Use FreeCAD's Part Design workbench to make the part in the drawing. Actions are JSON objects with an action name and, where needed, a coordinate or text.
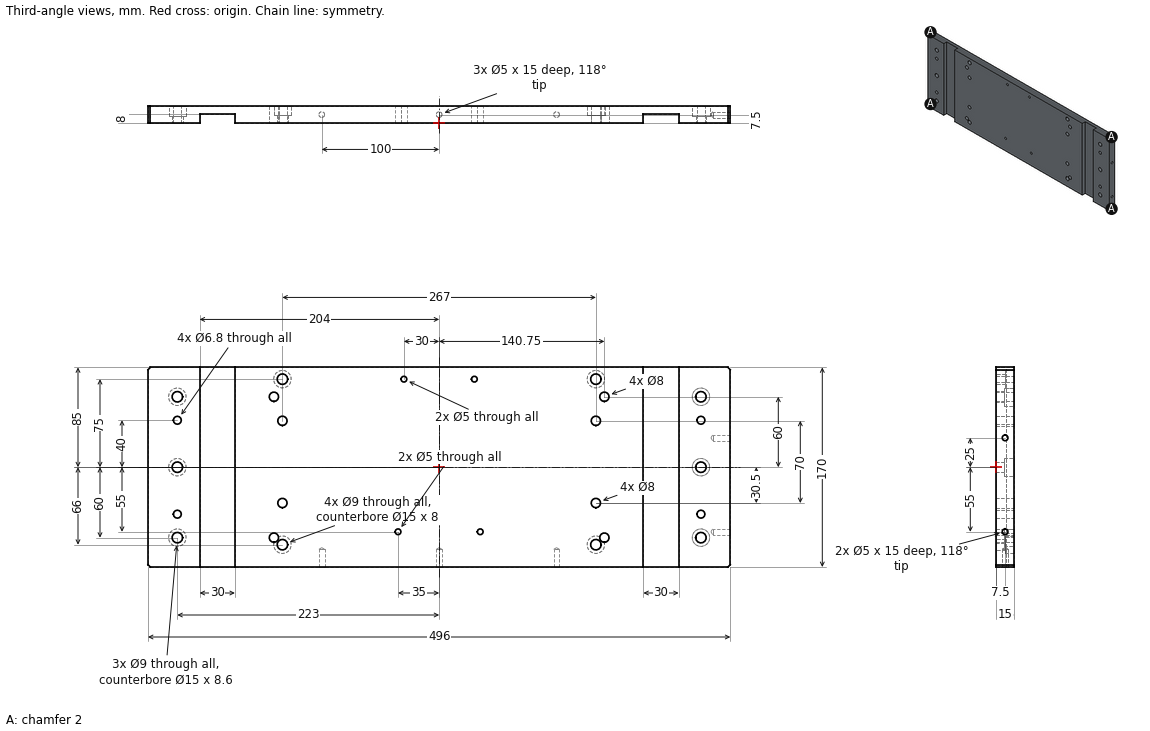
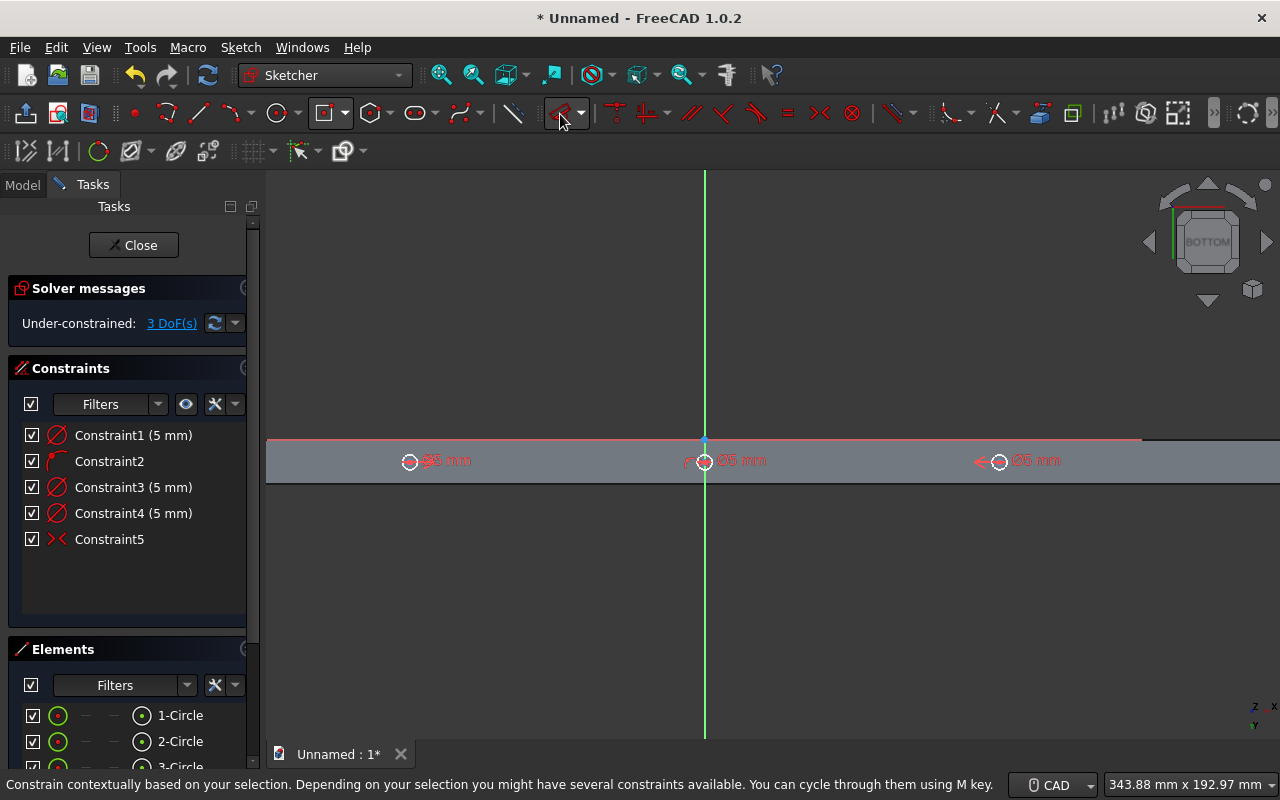
{"action": "scroll", "coordinate": [705, 462], "scroll_direction": "up", "scroll_amount": 3}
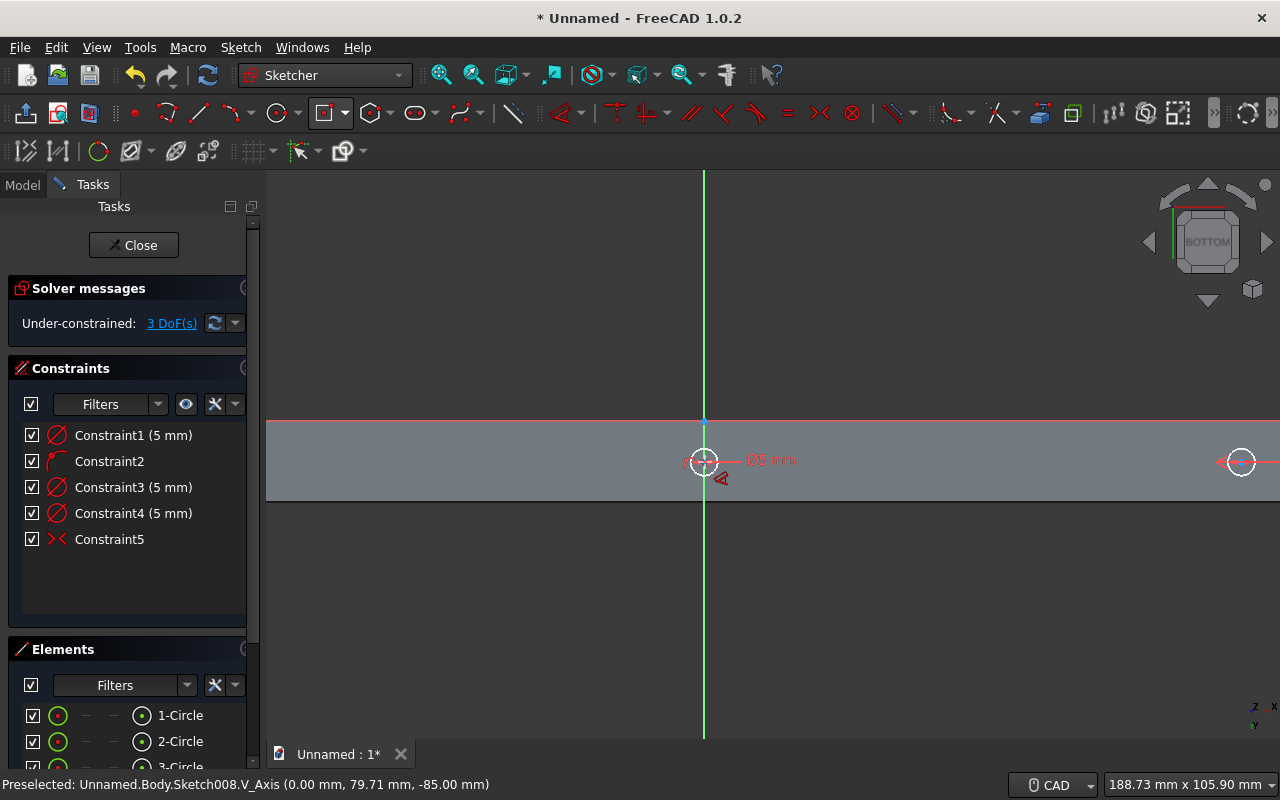
{"action": "left_click", "coordinate": [704, 462]}
{"action": "left_click", "coordinate": [738, 442]}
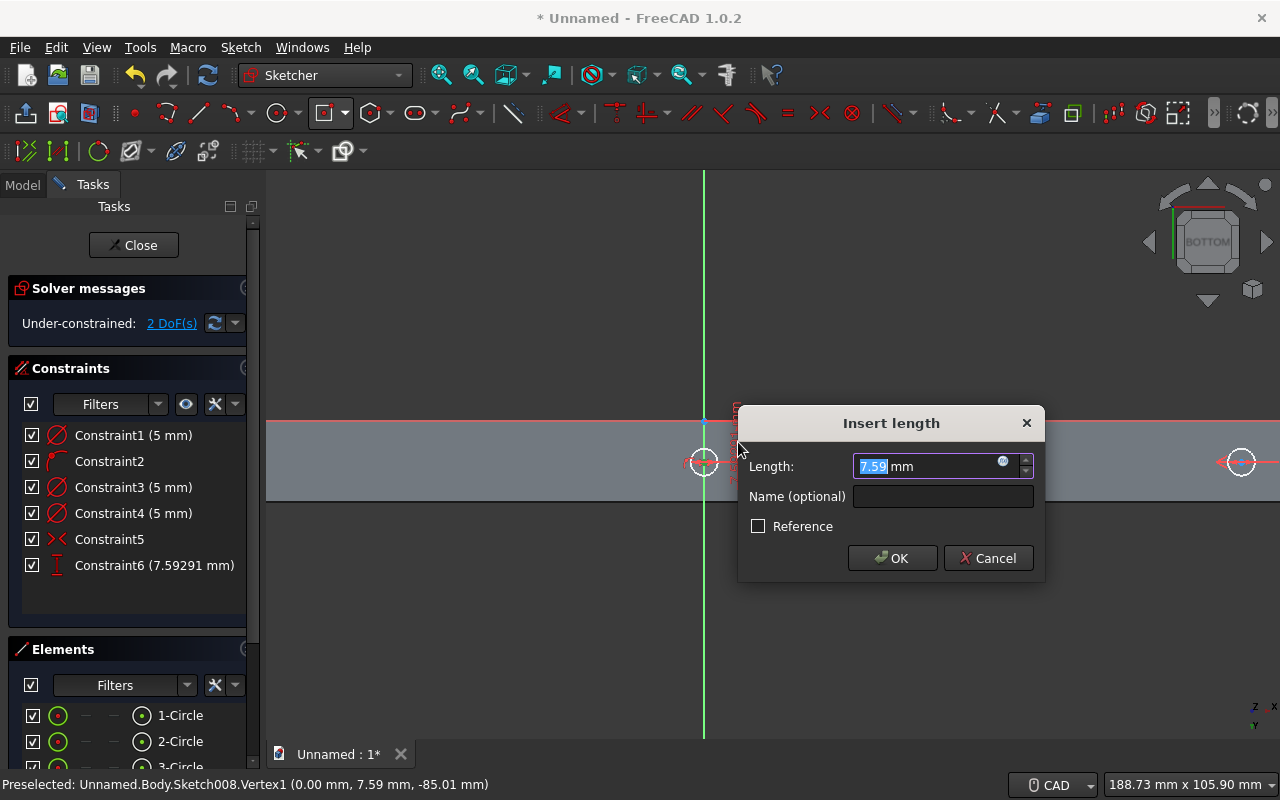
{"action": "type", "text": "7.5"}
{"action": "key", "text": "Return"}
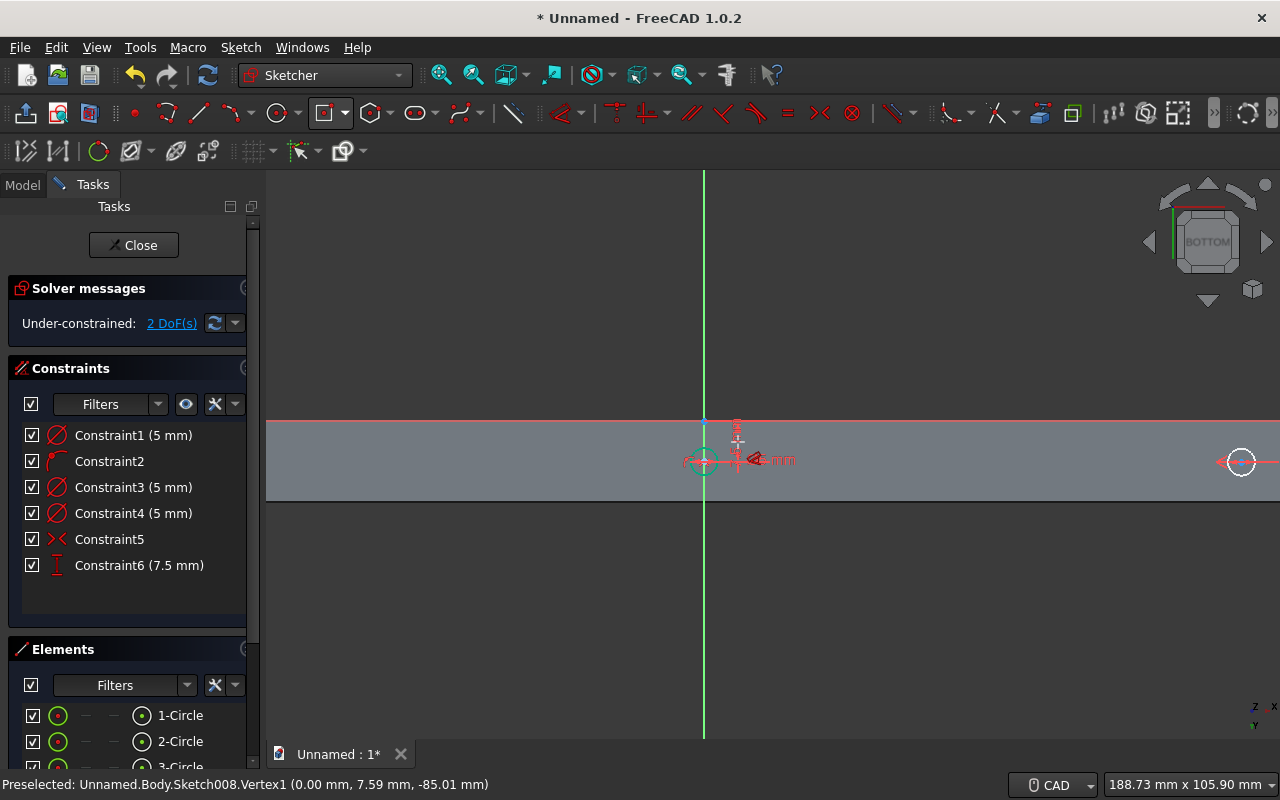
{"action": "scroll", "coordinate": [705, 462], "scroll_direction": "down", "scroll_amount": 3}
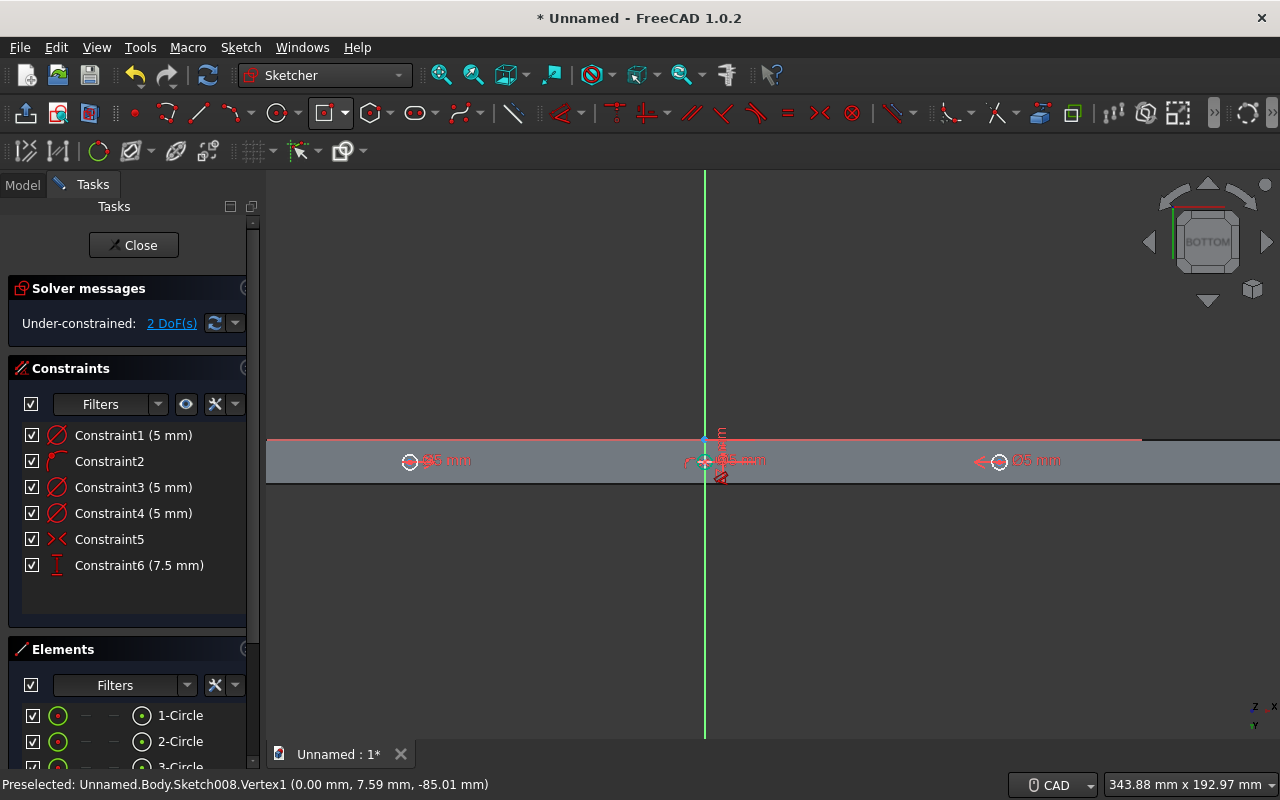
{"action": "left_click", "coordinate": [410, 462]}
{"action": "left_click", "coordinate": [557, 406]}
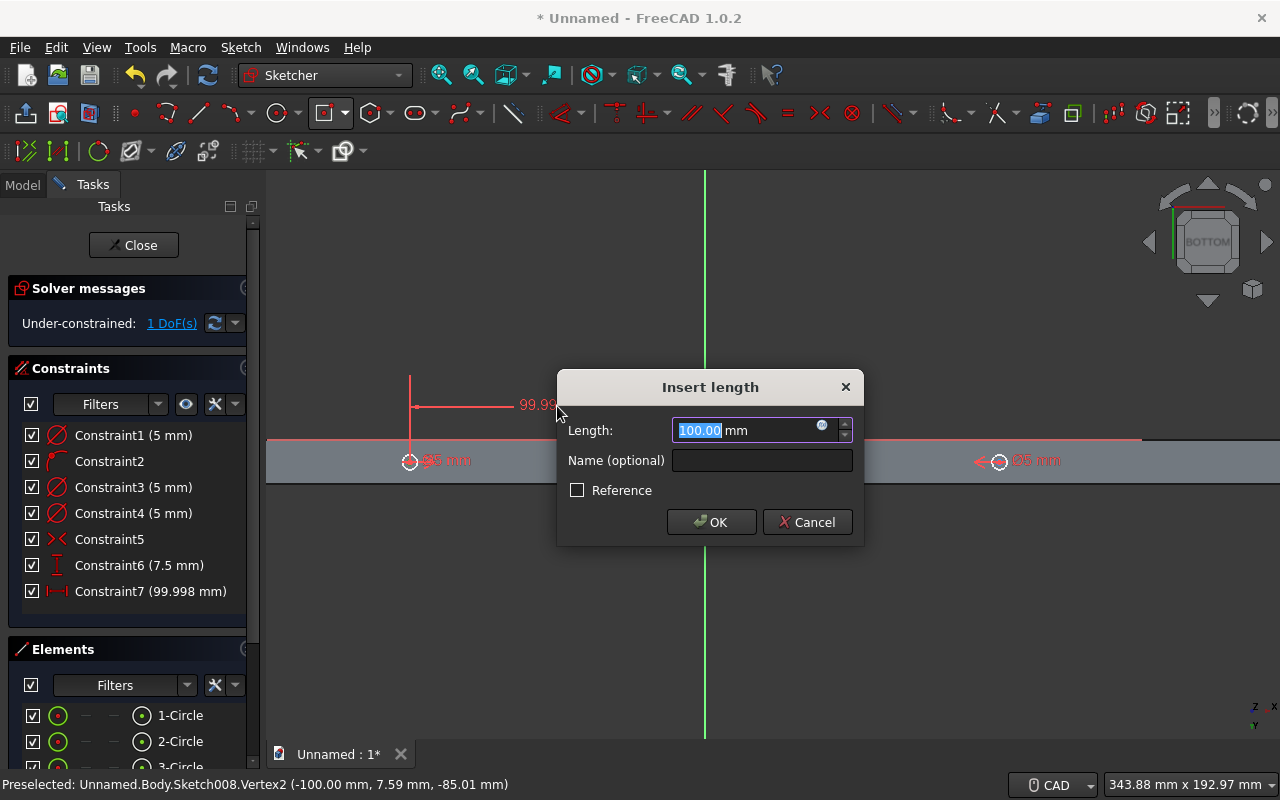
{"action": "type", "text": "100"}
{"action": "key", "text": "Return"}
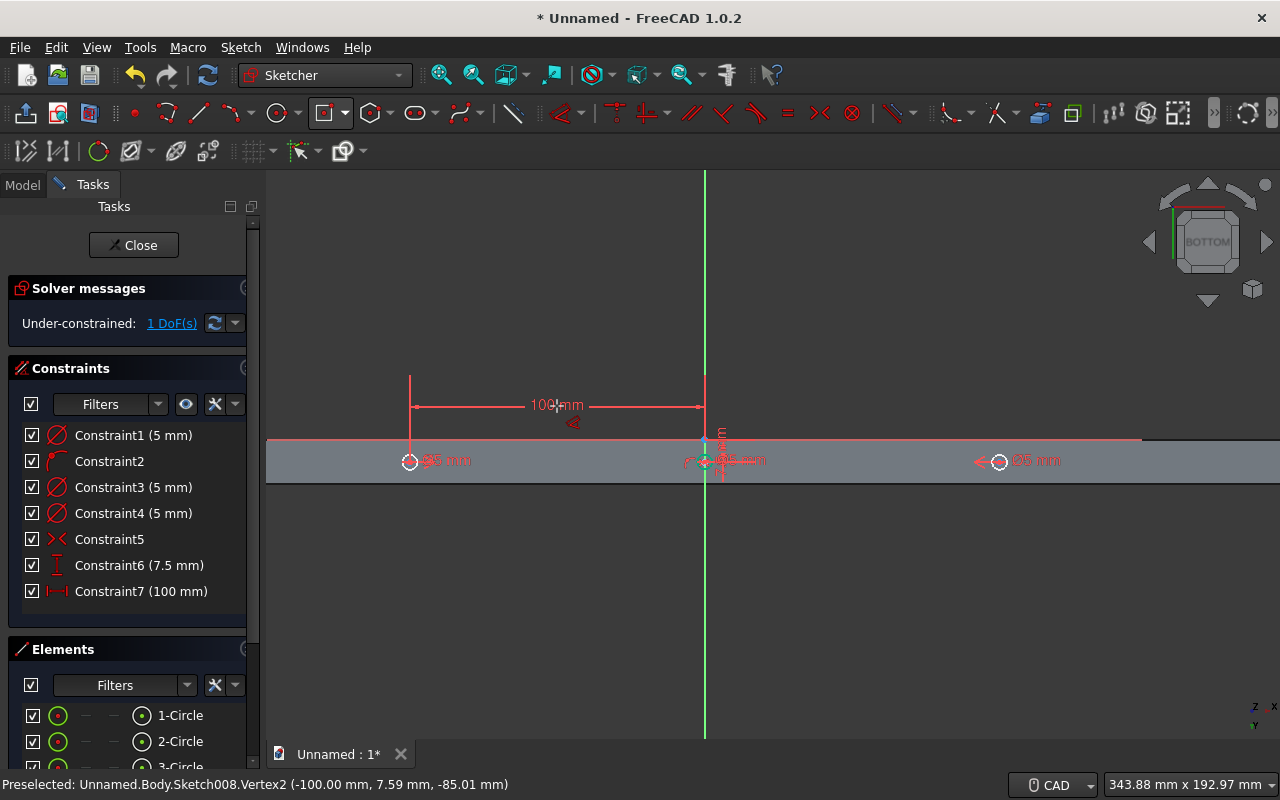
{"action": "scroll", "coordinate": [410, 462], "scroll_direction": "up", "scroll_amount": 3}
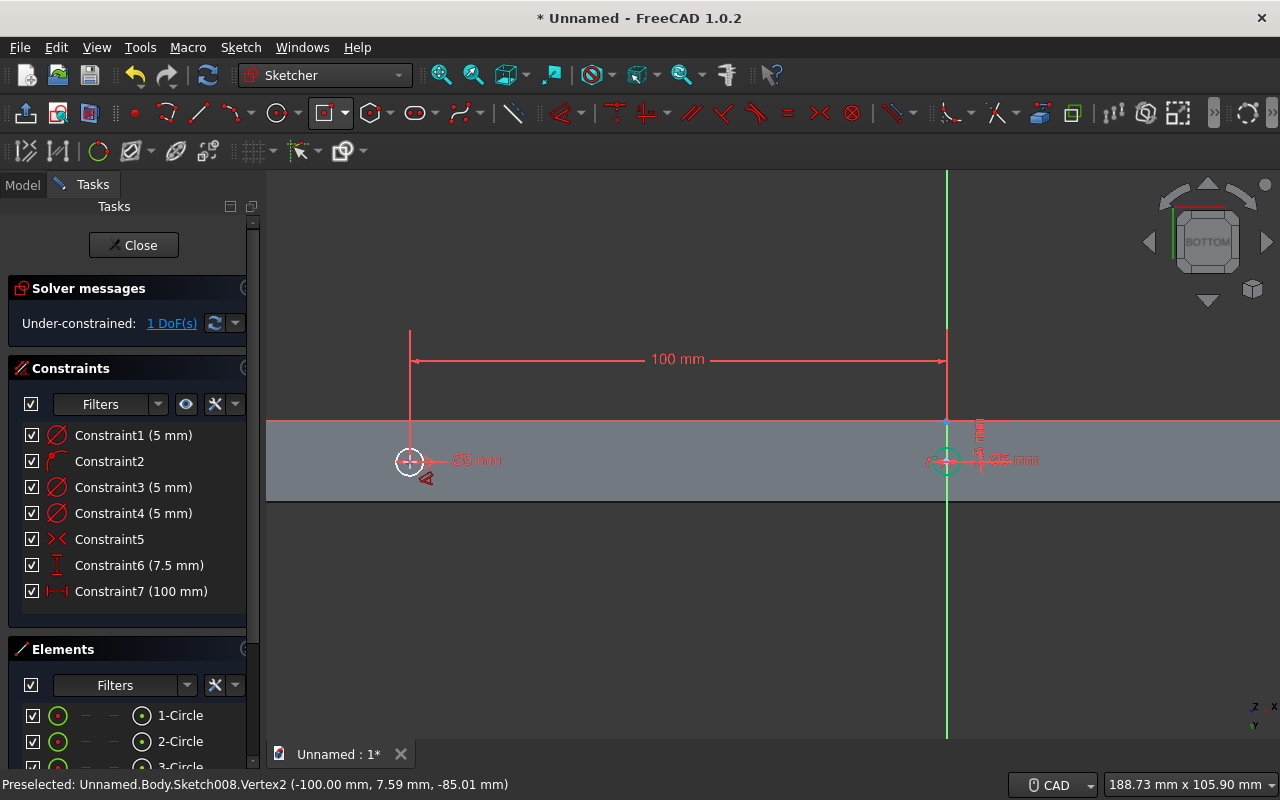
{"action": "left_click", "coordinate": [410, 462]}
{"action": "left_click", "coordinate": [376, 442]}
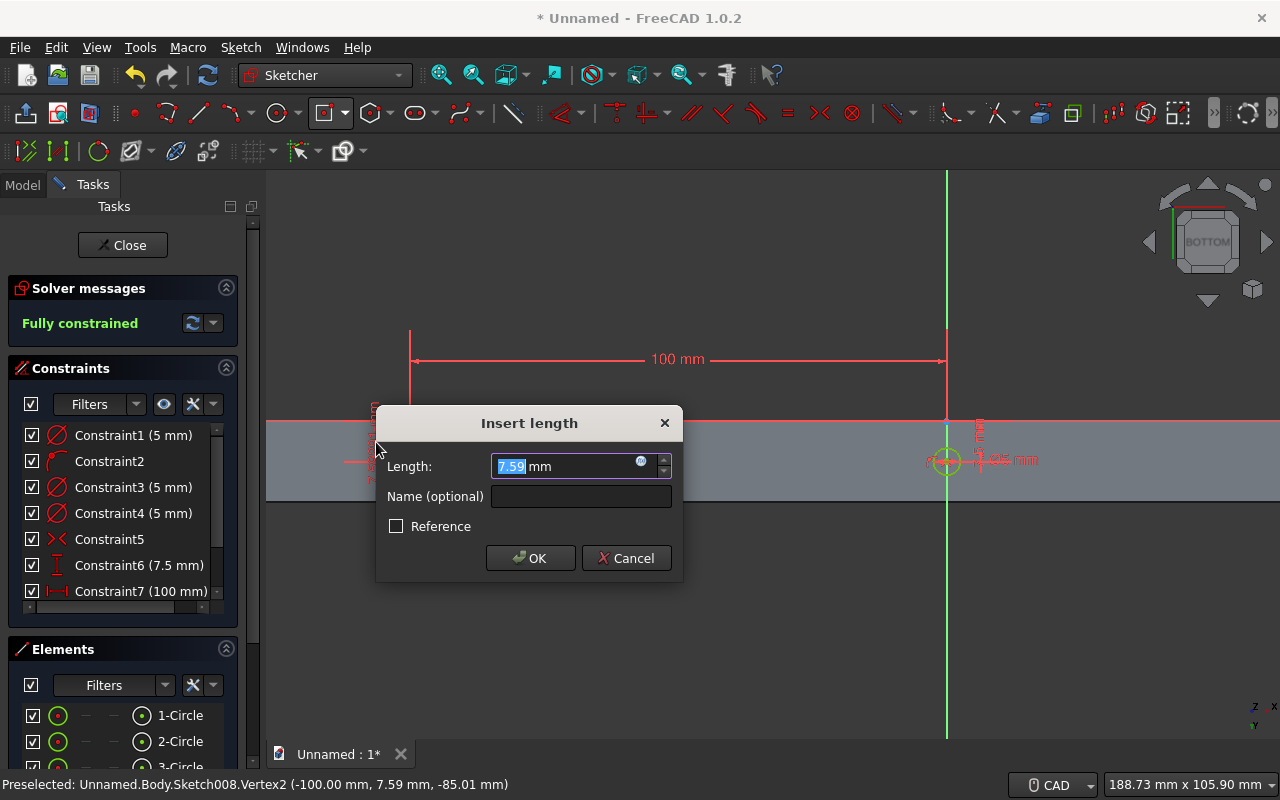
{"action": "type", "text": "7.5"}
{"action": "key", "text": "Return"}
{"action": "key", "text": "Escape"}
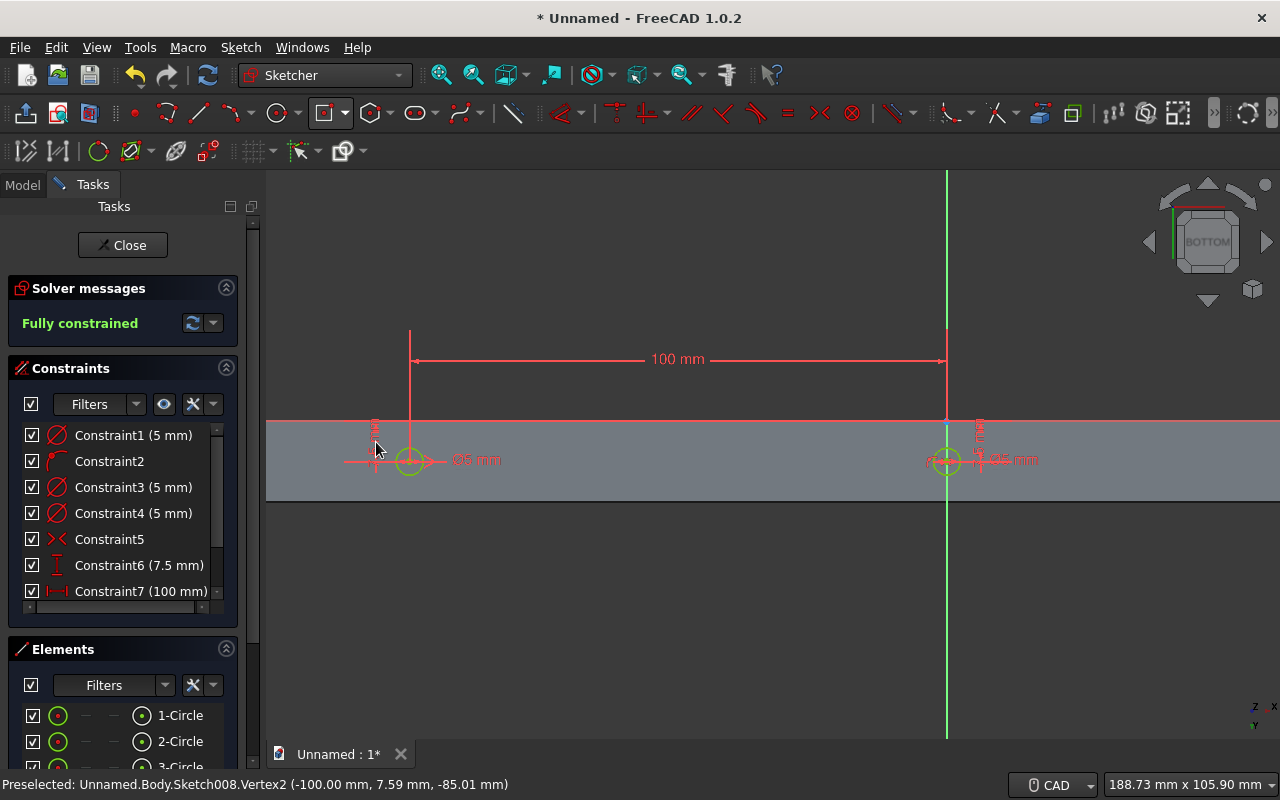
{"action": "left_click", "coordinate": [123, 245]}